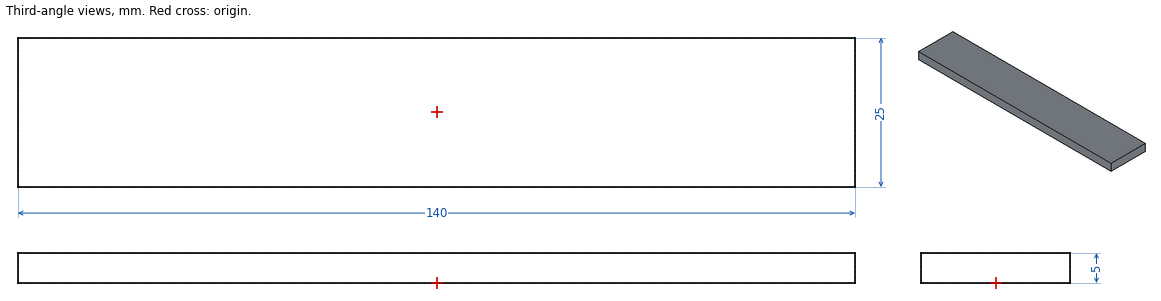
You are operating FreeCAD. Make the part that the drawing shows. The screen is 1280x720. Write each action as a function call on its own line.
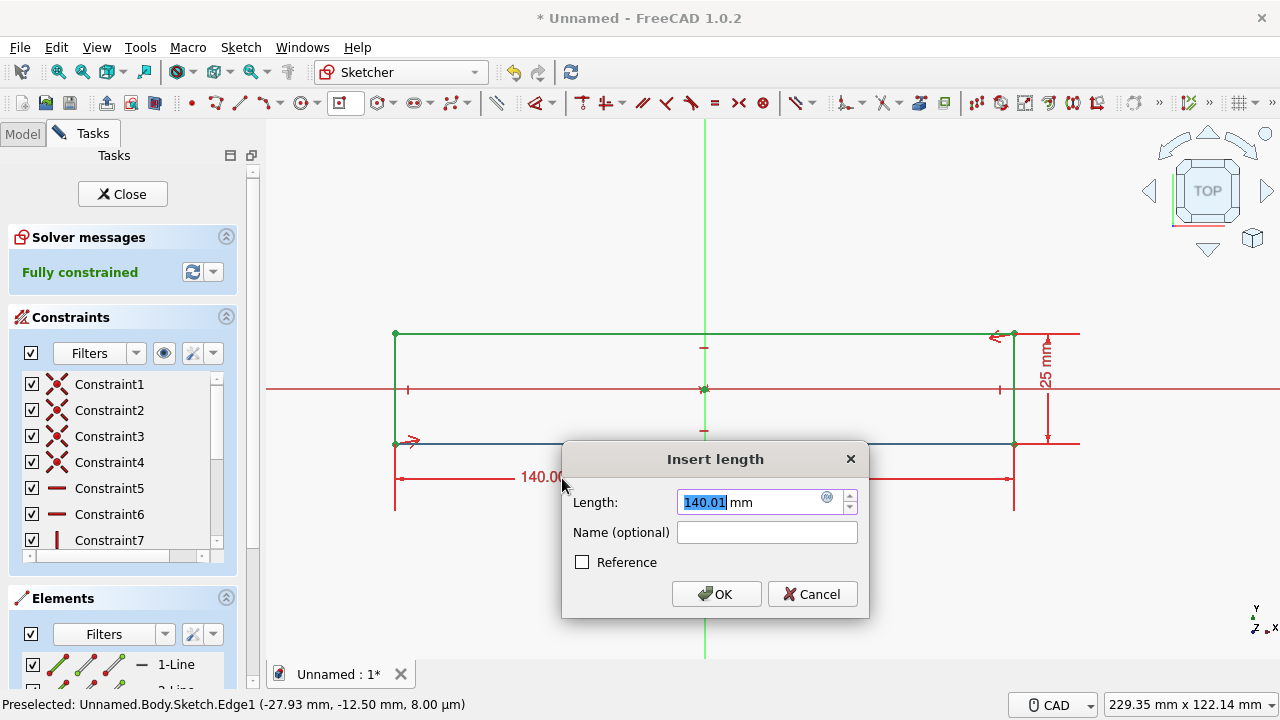
text(140)
key(Return)
key(Escape)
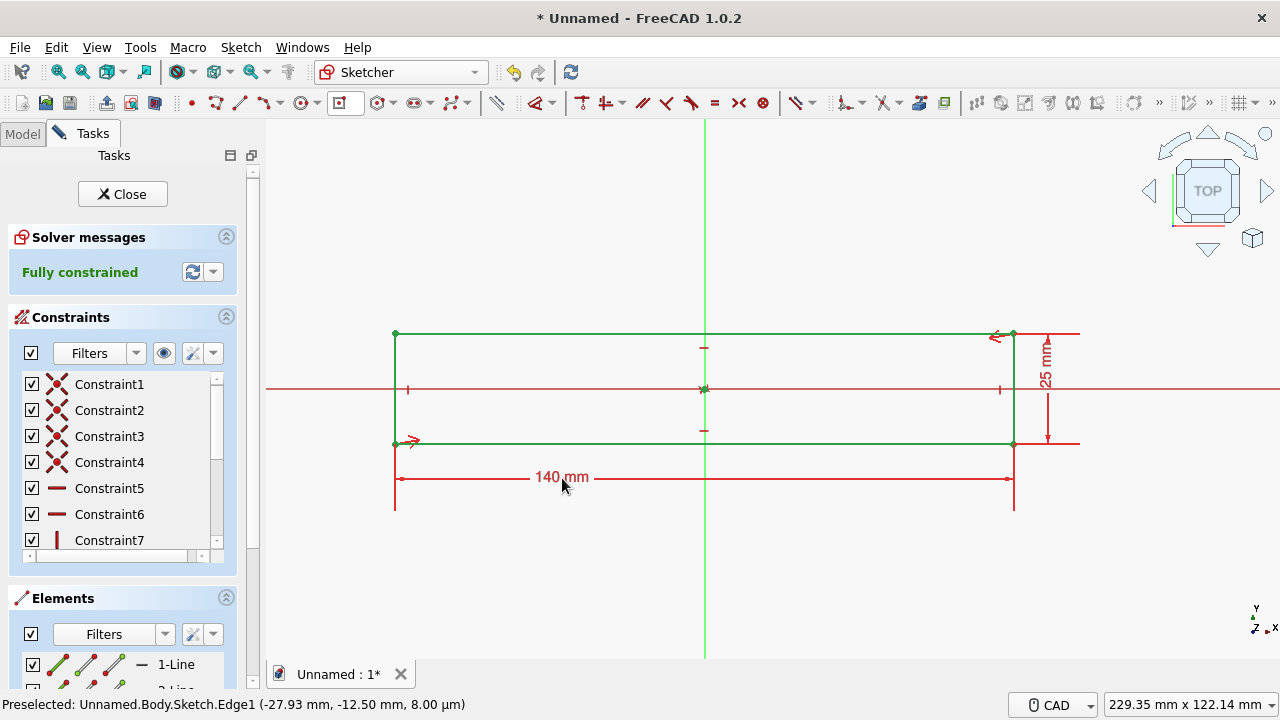
click(123, 194)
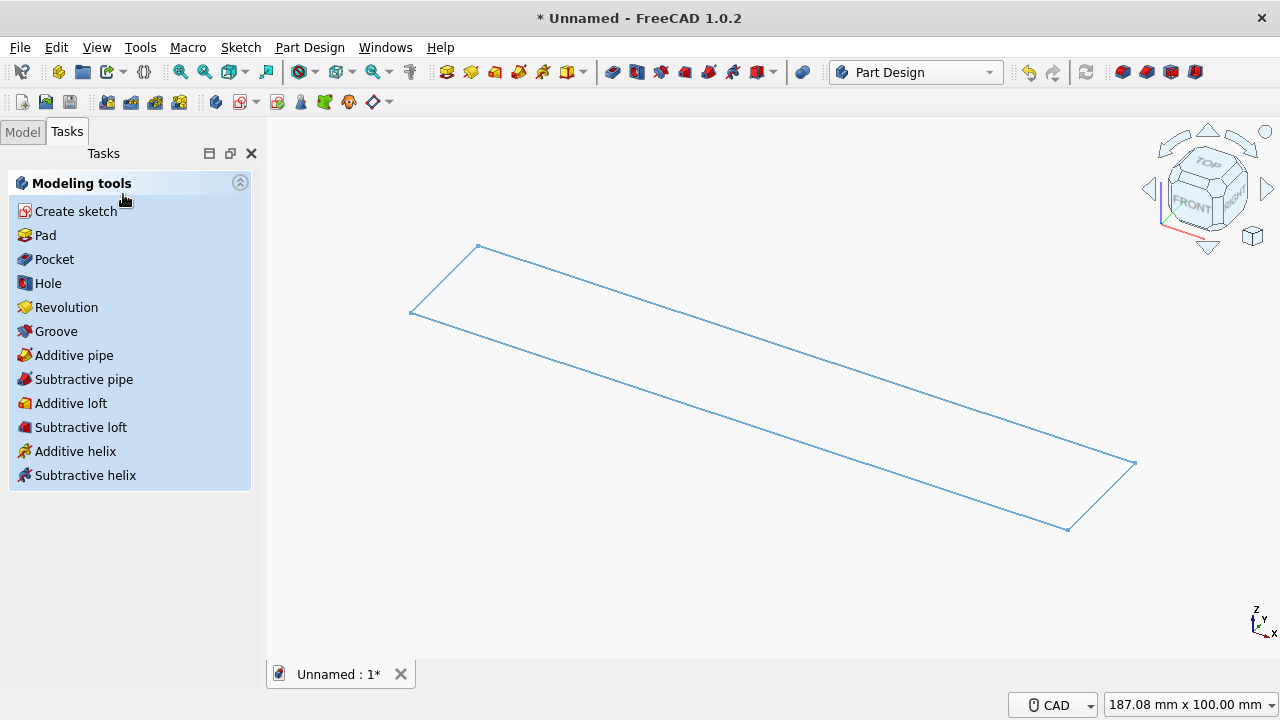
click(448, 72)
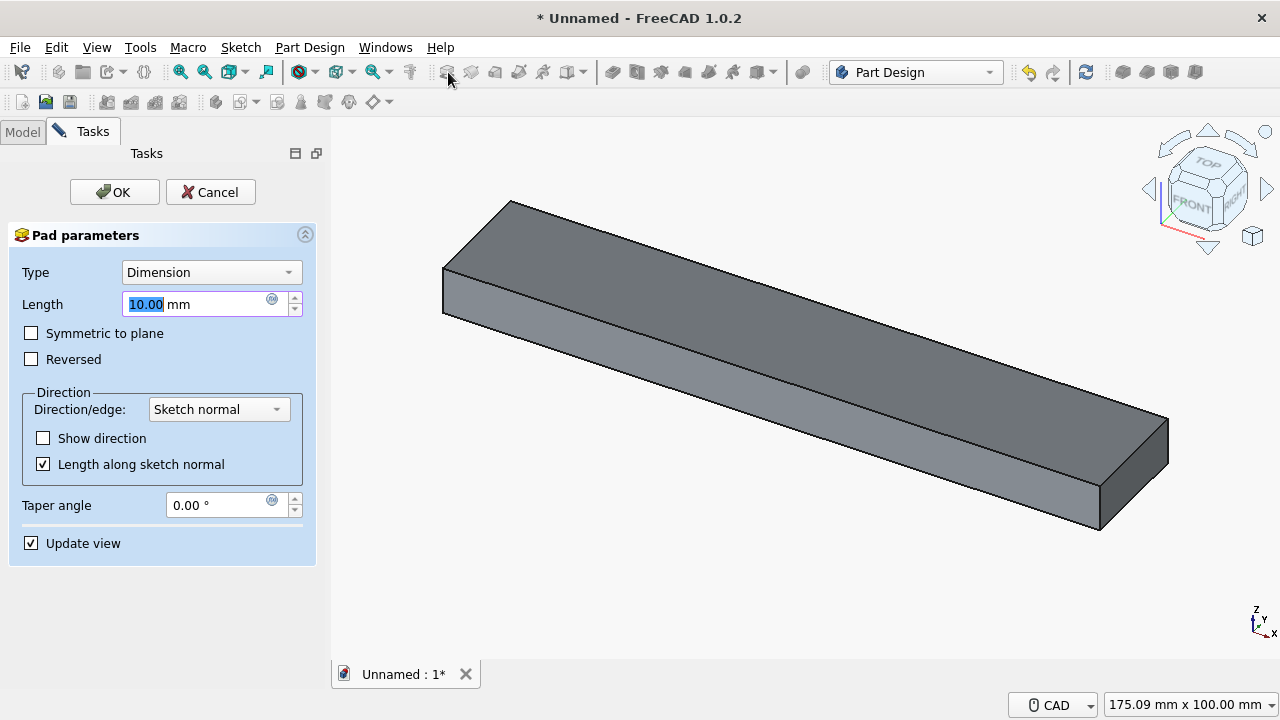
text(5)
key(Tab)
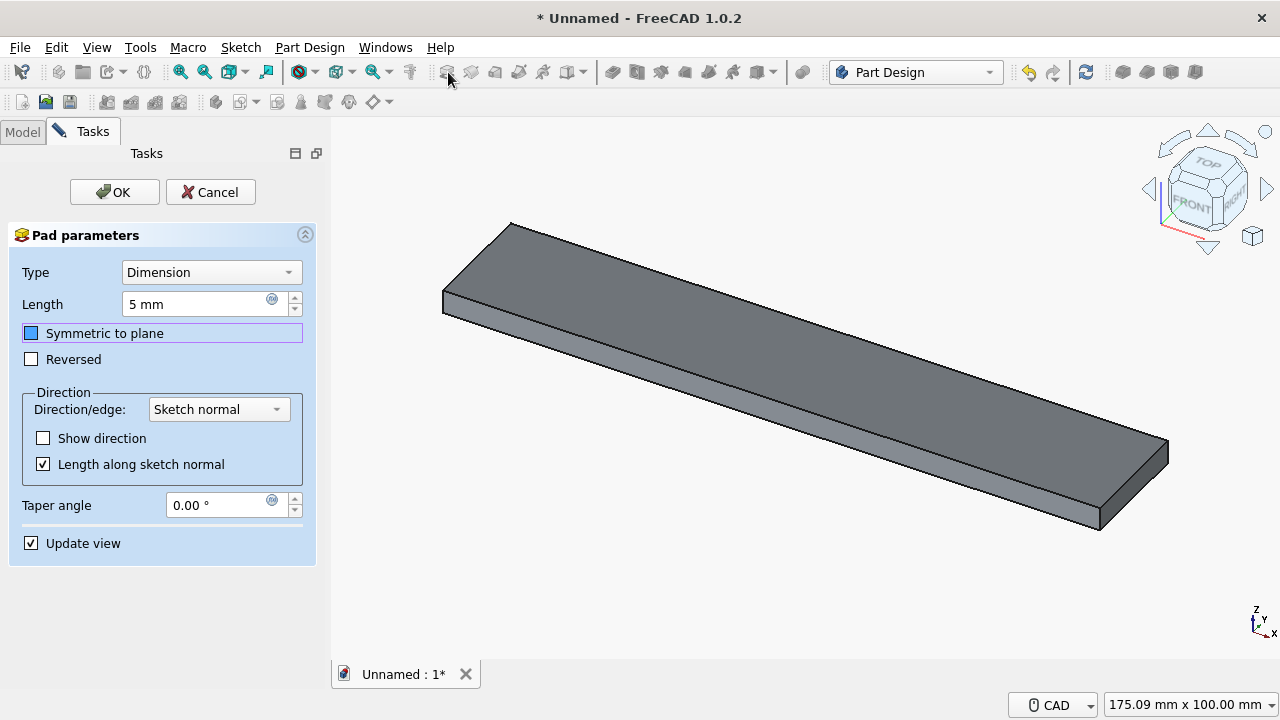
click(115, 192)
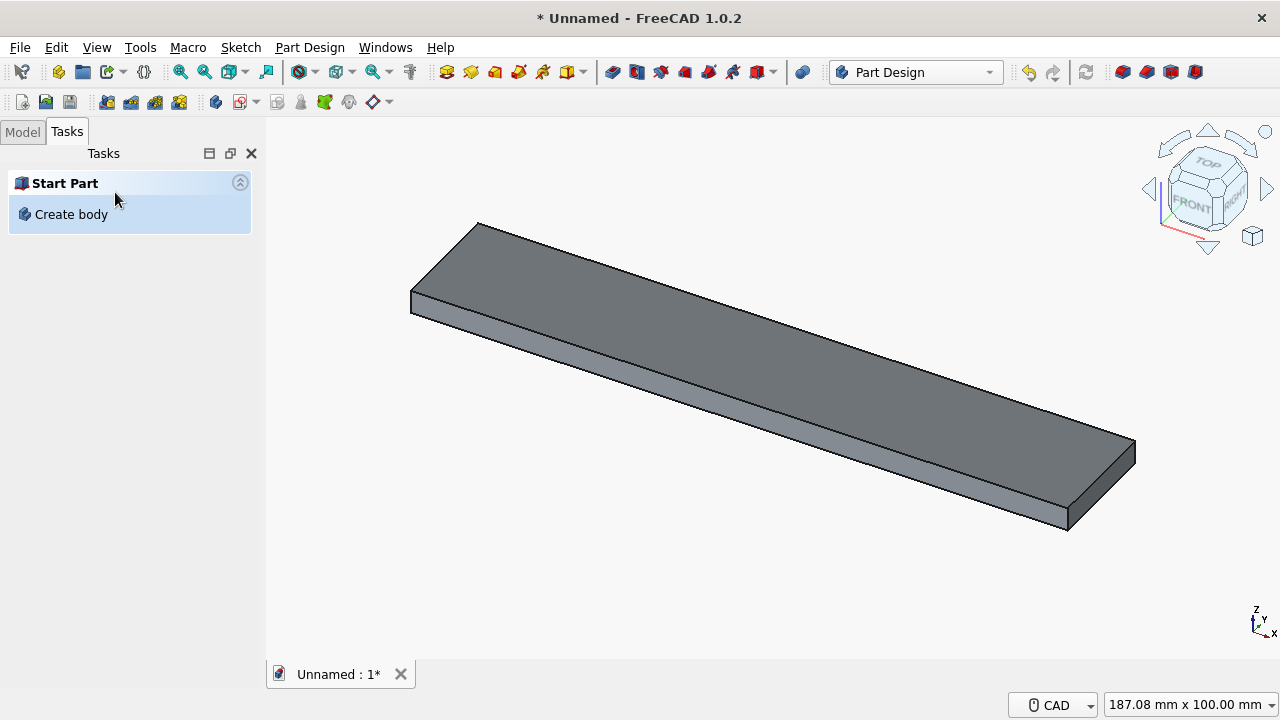
key(0)